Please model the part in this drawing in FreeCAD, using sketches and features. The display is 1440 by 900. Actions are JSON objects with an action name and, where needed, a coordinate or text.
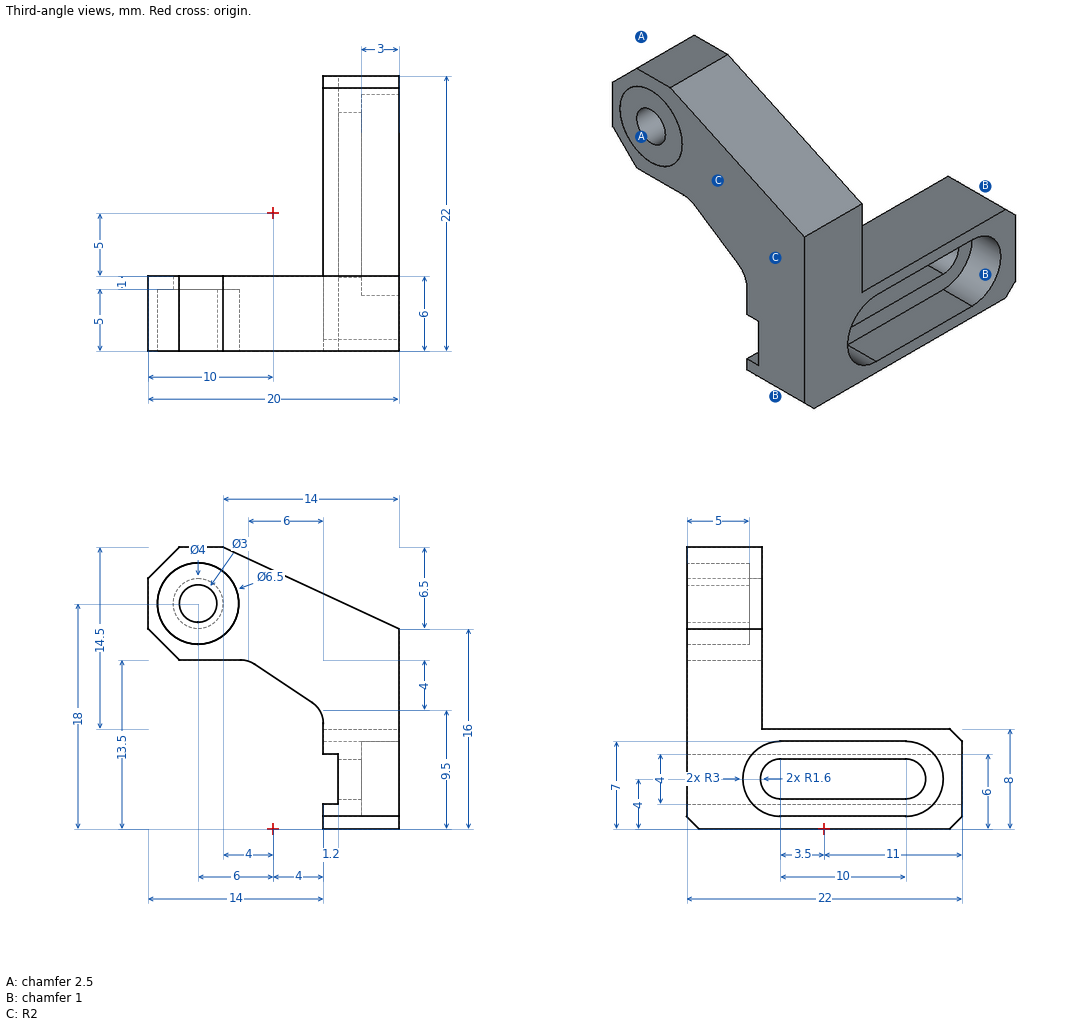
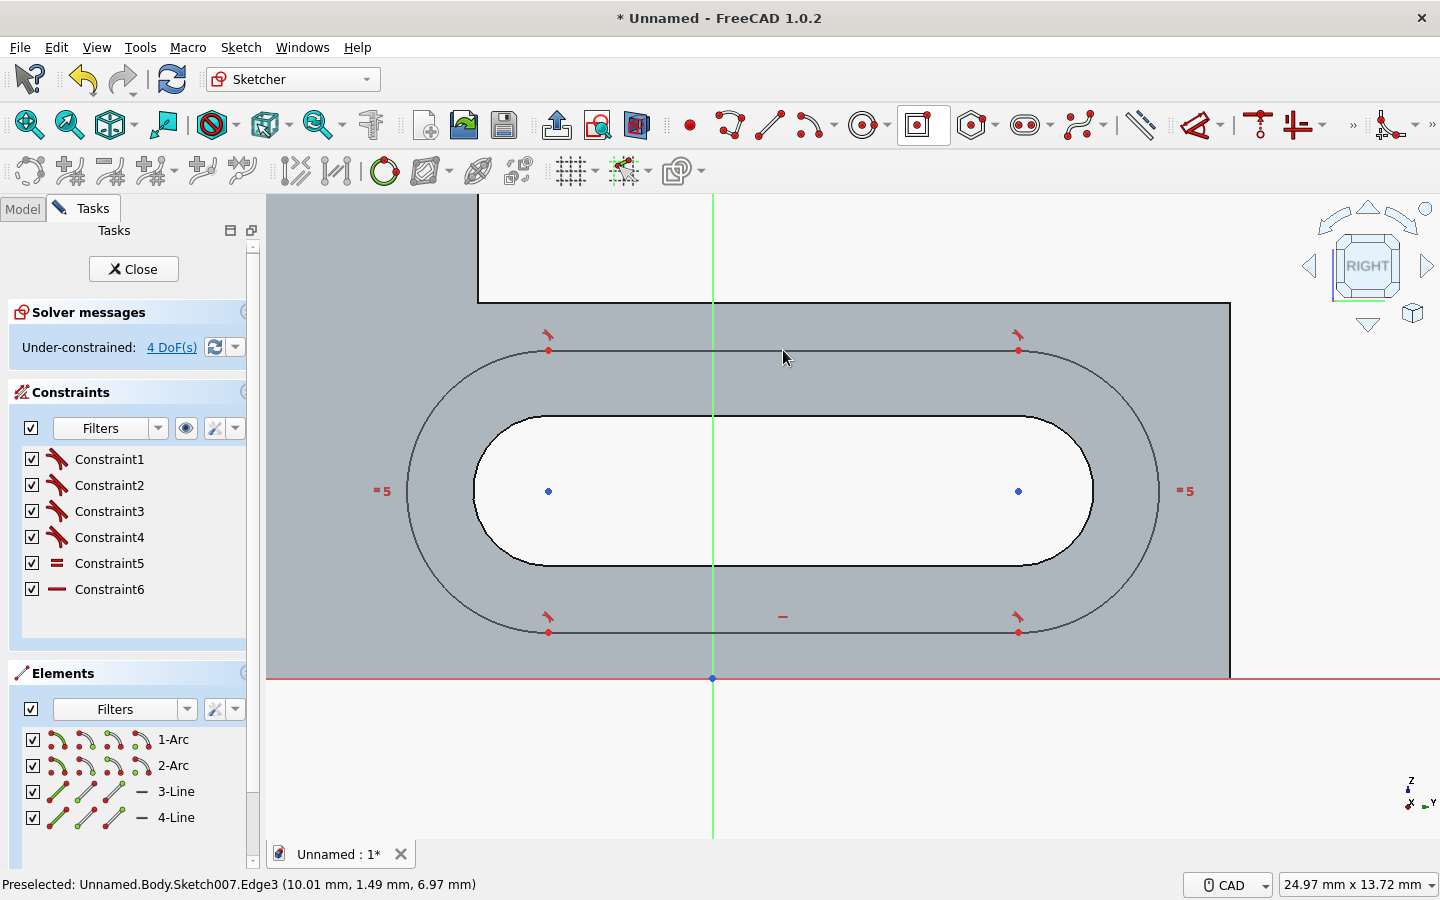
{"action": "left_click", "coordinate": [1196, 126]}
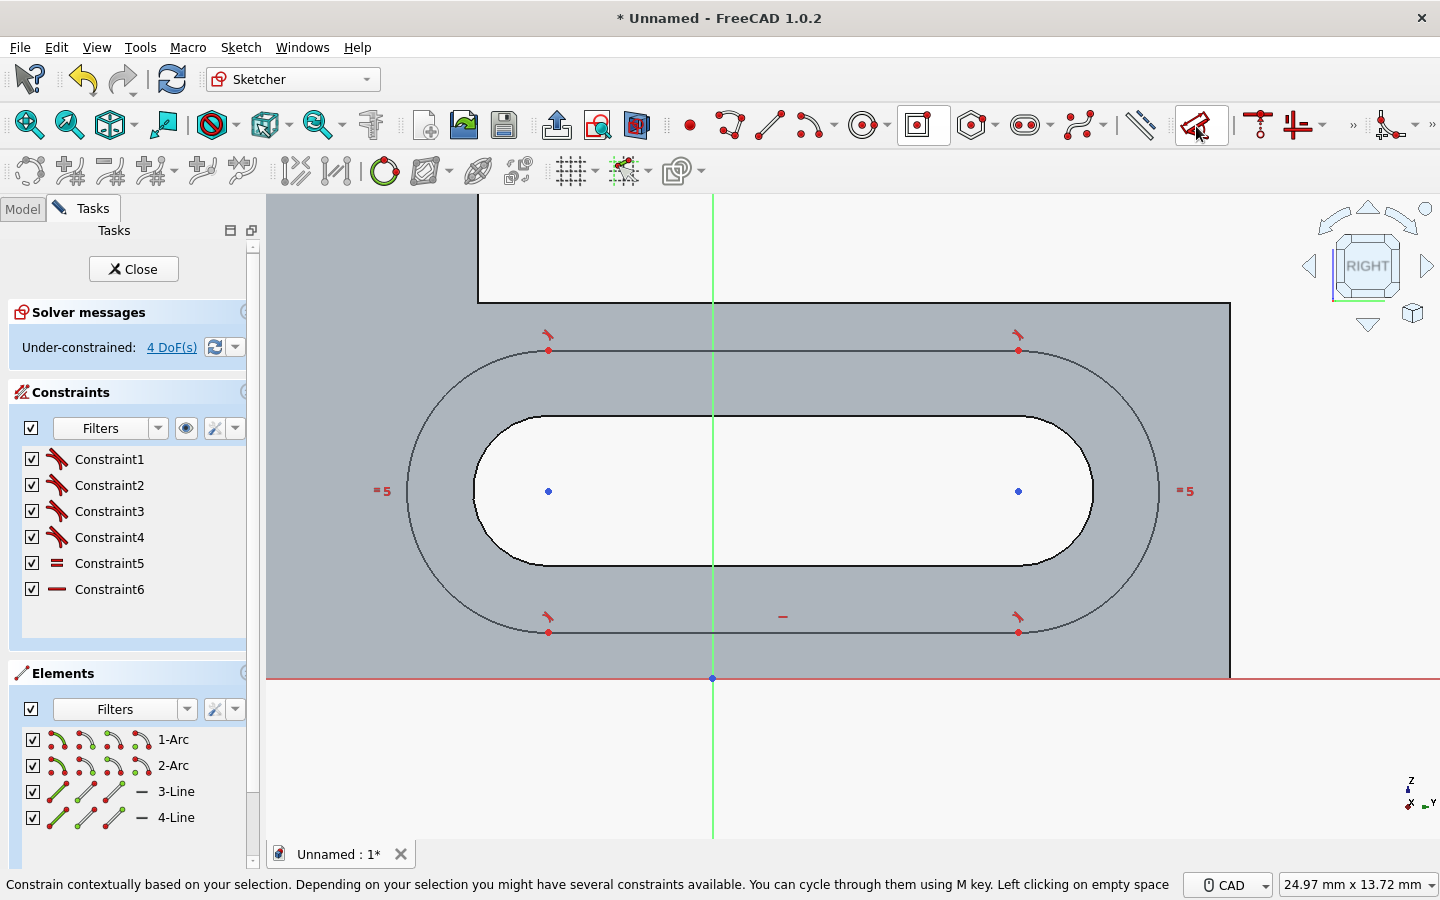
{"action": "left_click", "coordinate": [434, 409]}
{"action": "left_click", "coordinate": [408, 390]}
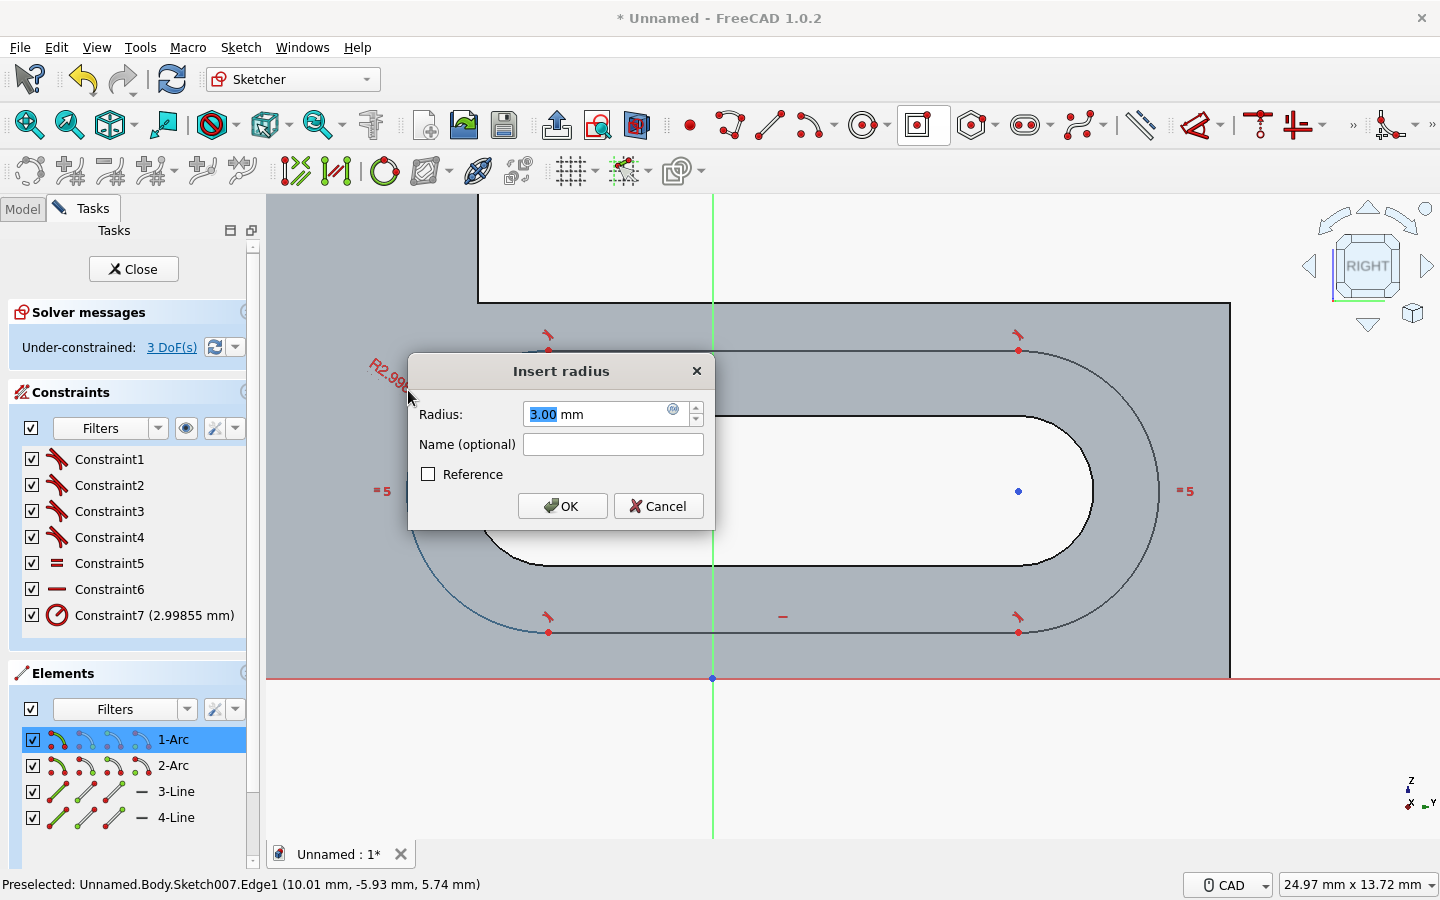
{"action": "type", "text": "3"}
{"action": "key", "text": "Return"}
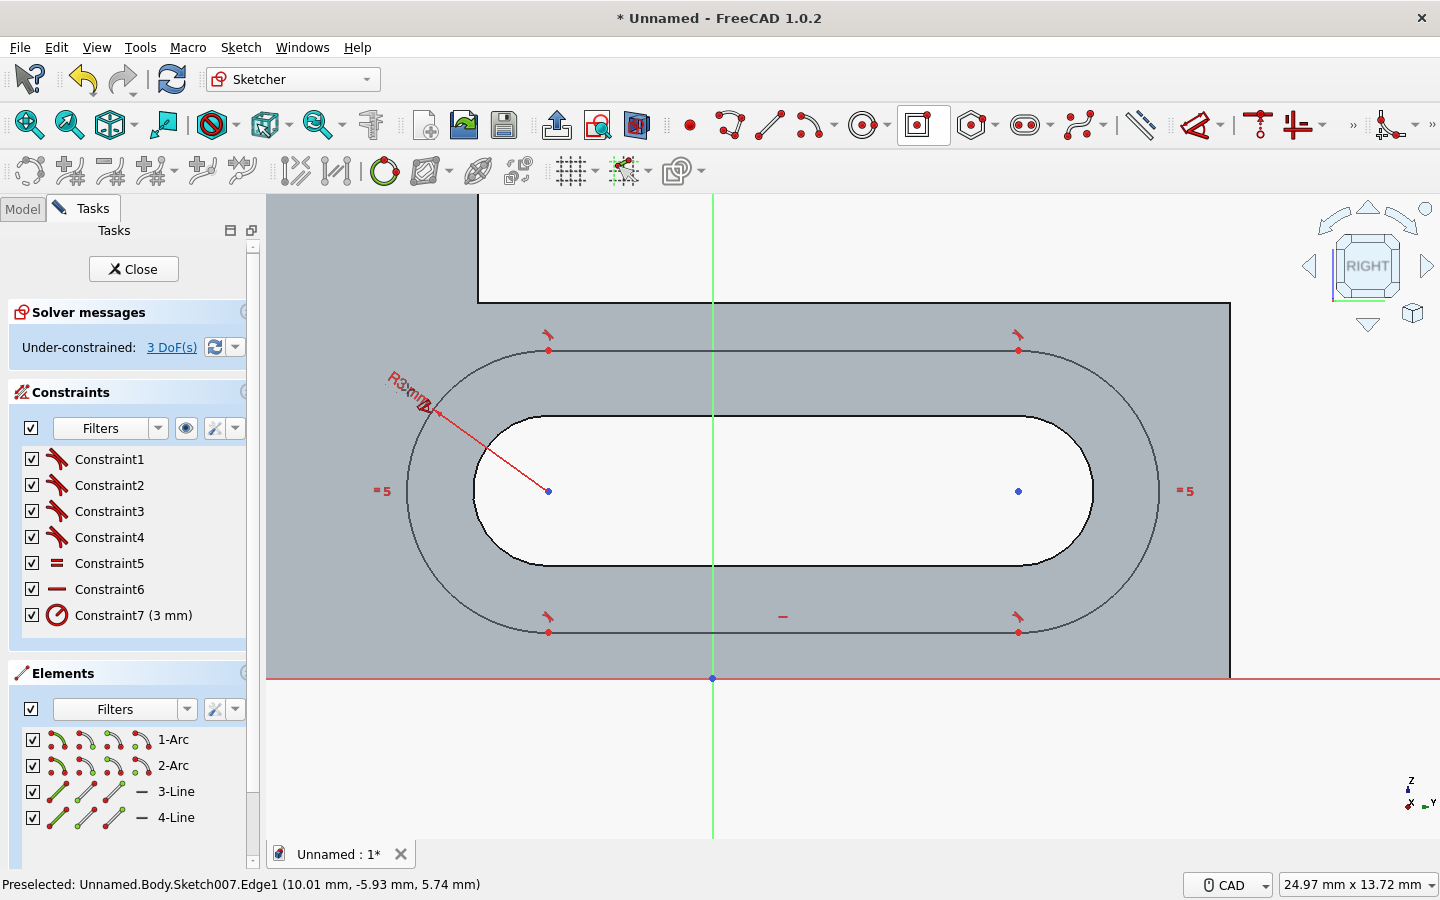
{"action": "left_click", "coordinate": [689, 351]}
{"action": "left_click", "coordinate": [783, 317]}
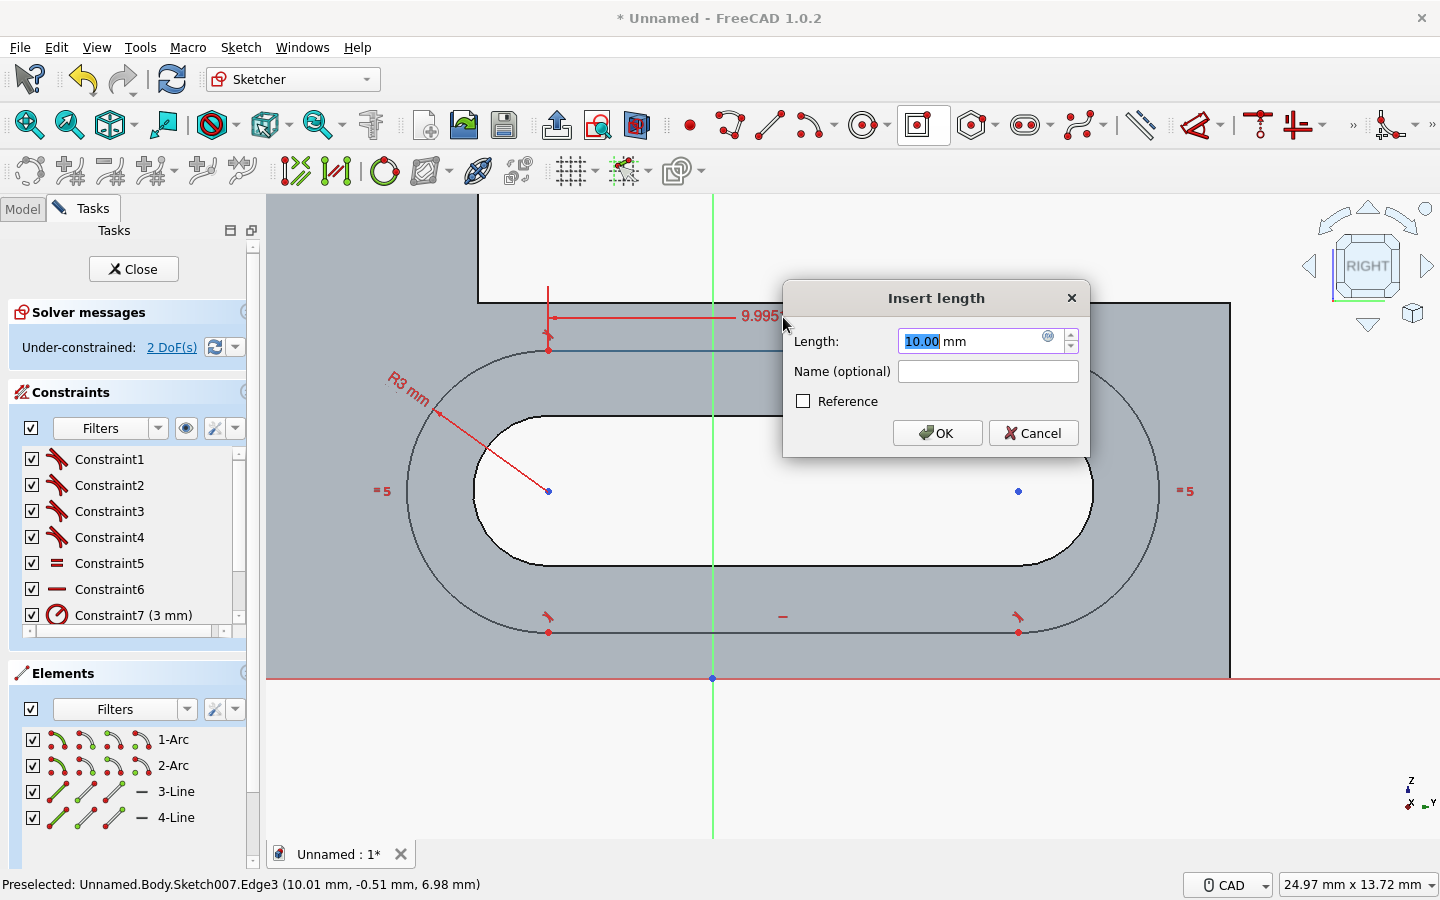
{"action": "type", "text": "10"}
{"action": "key", "text": "Return"}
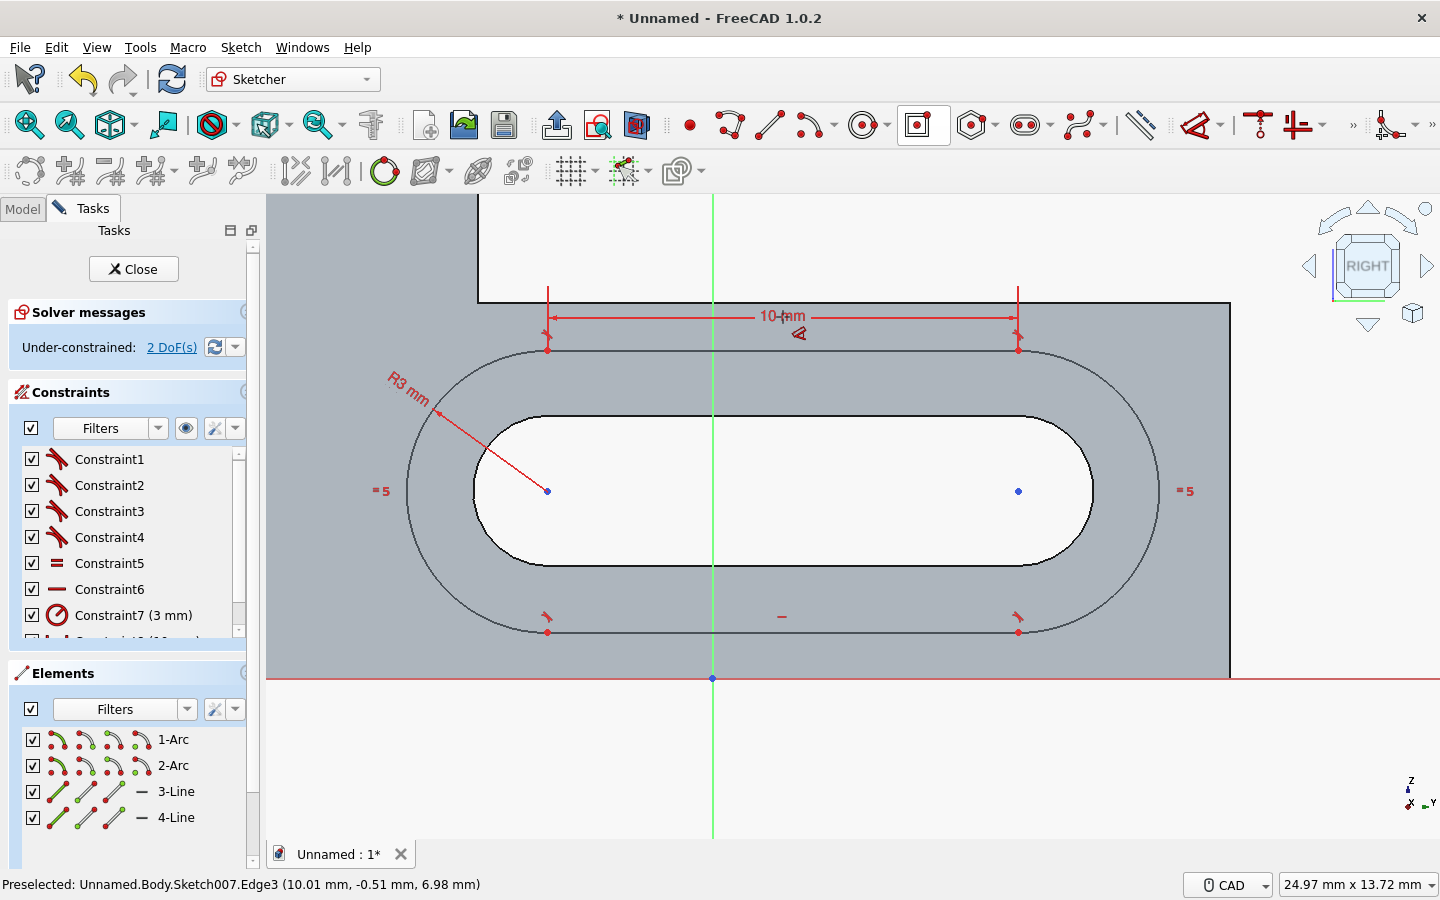
{"action": "left_click", "coordinate": [548, 351]}
{"action": "left_click", "coordinate": [514, 515]}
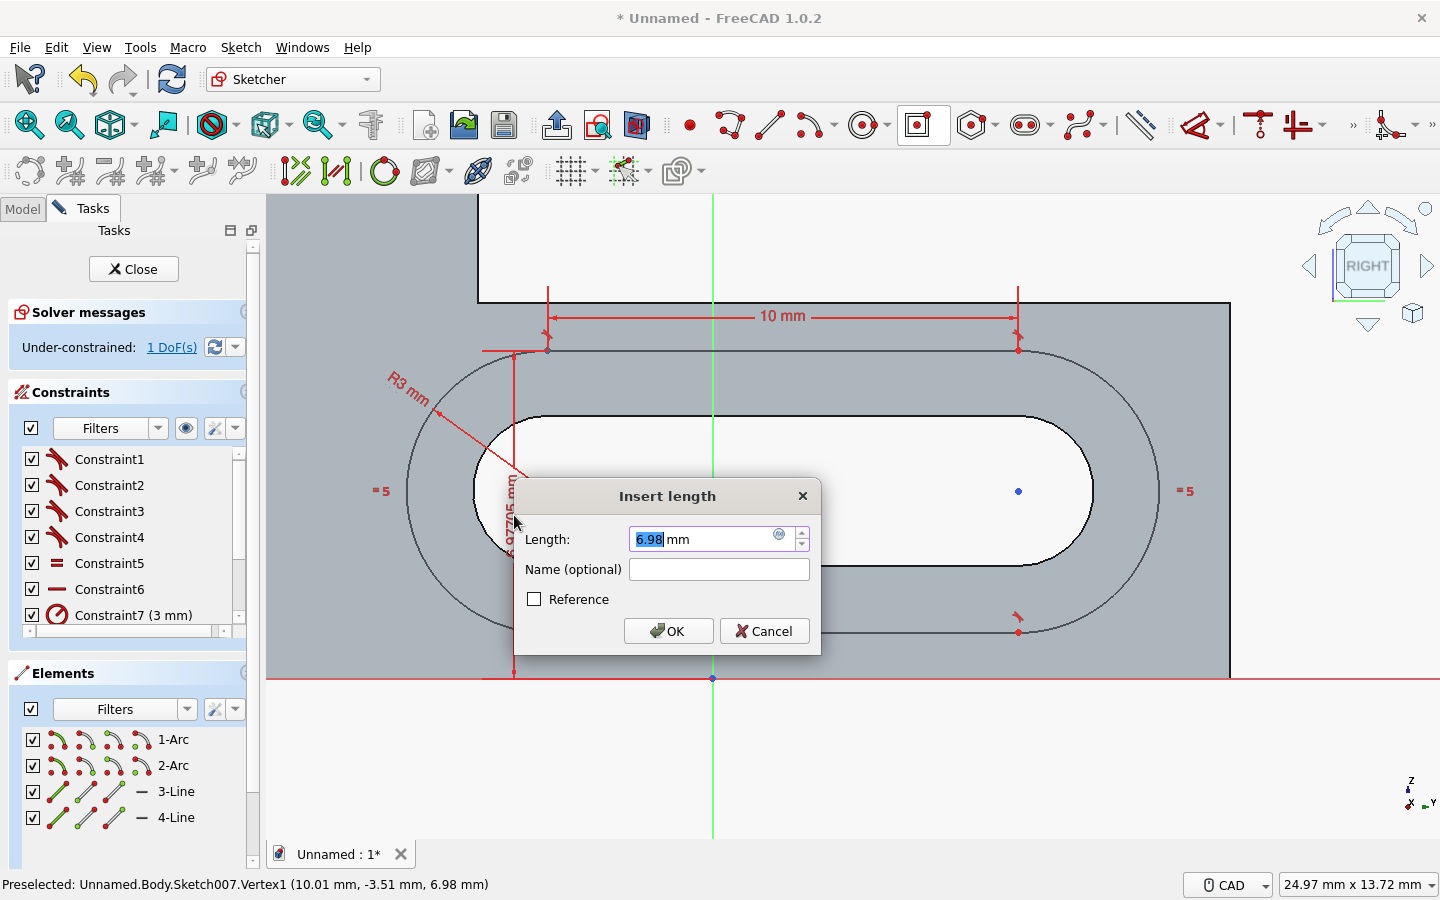
{"action": "type", "text": "7"}
{"action": "key", "text": "Return"}